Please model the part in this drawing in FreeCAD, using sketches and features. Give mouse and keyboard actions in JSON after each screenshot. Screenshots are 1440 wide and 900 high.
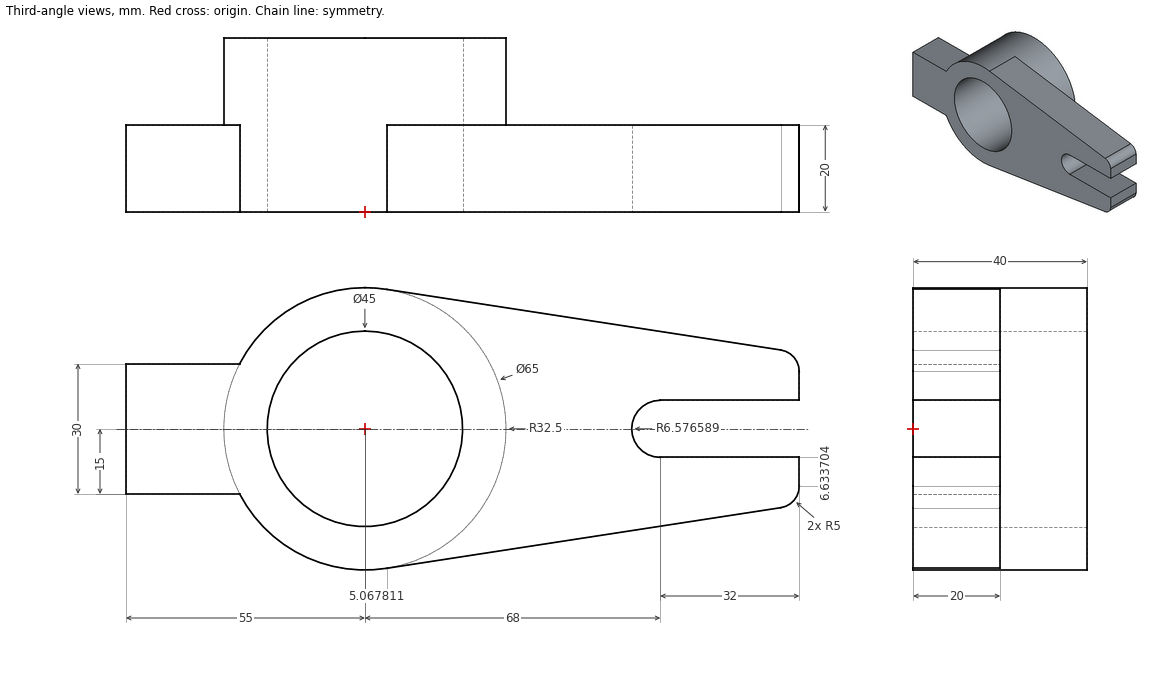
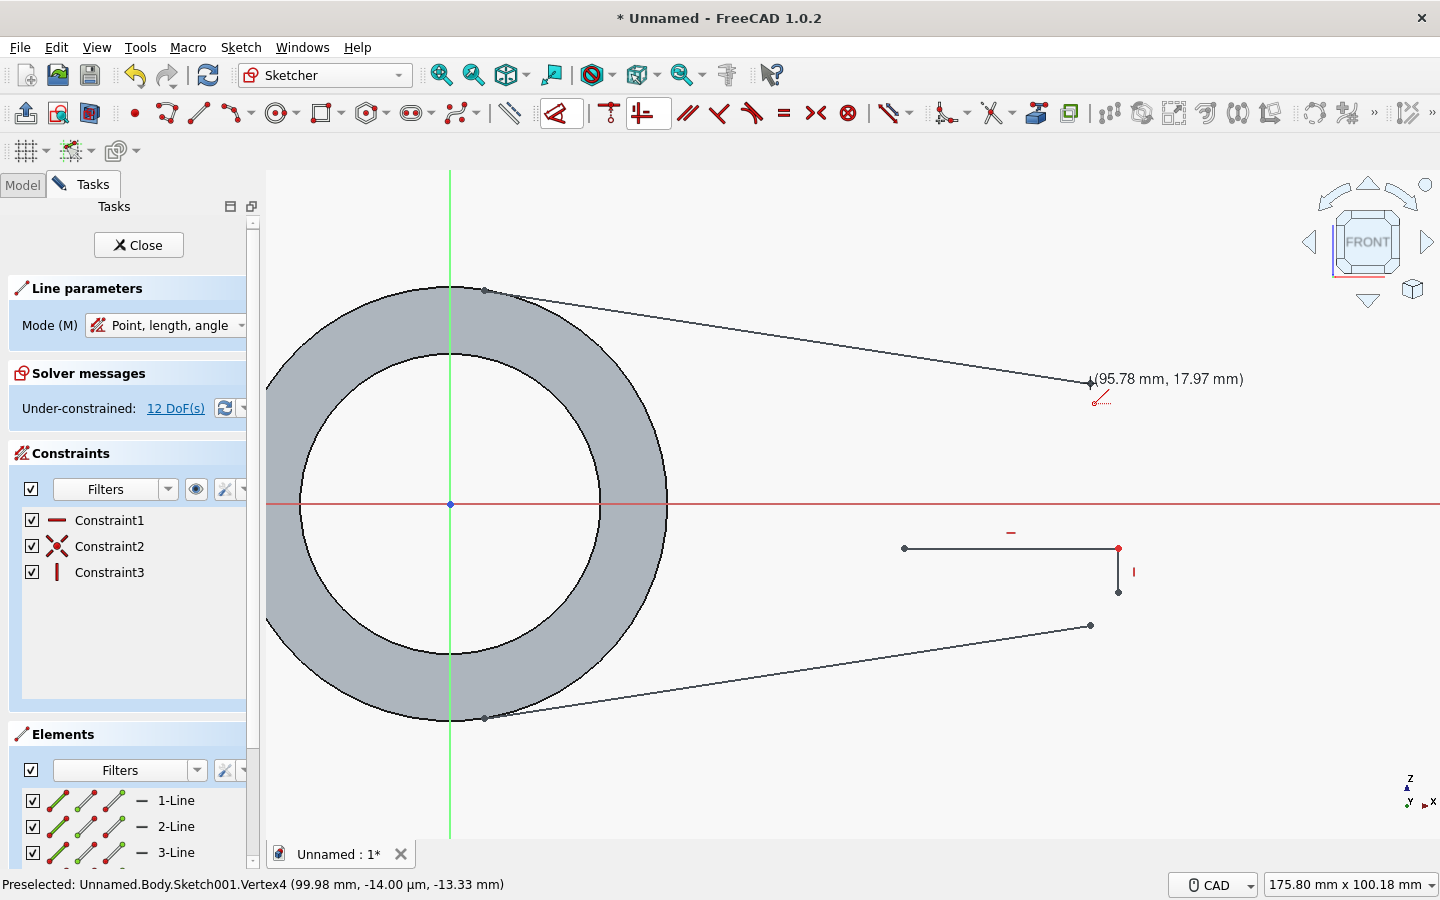
{"action": "left_click", "coordinate": [168, 114]}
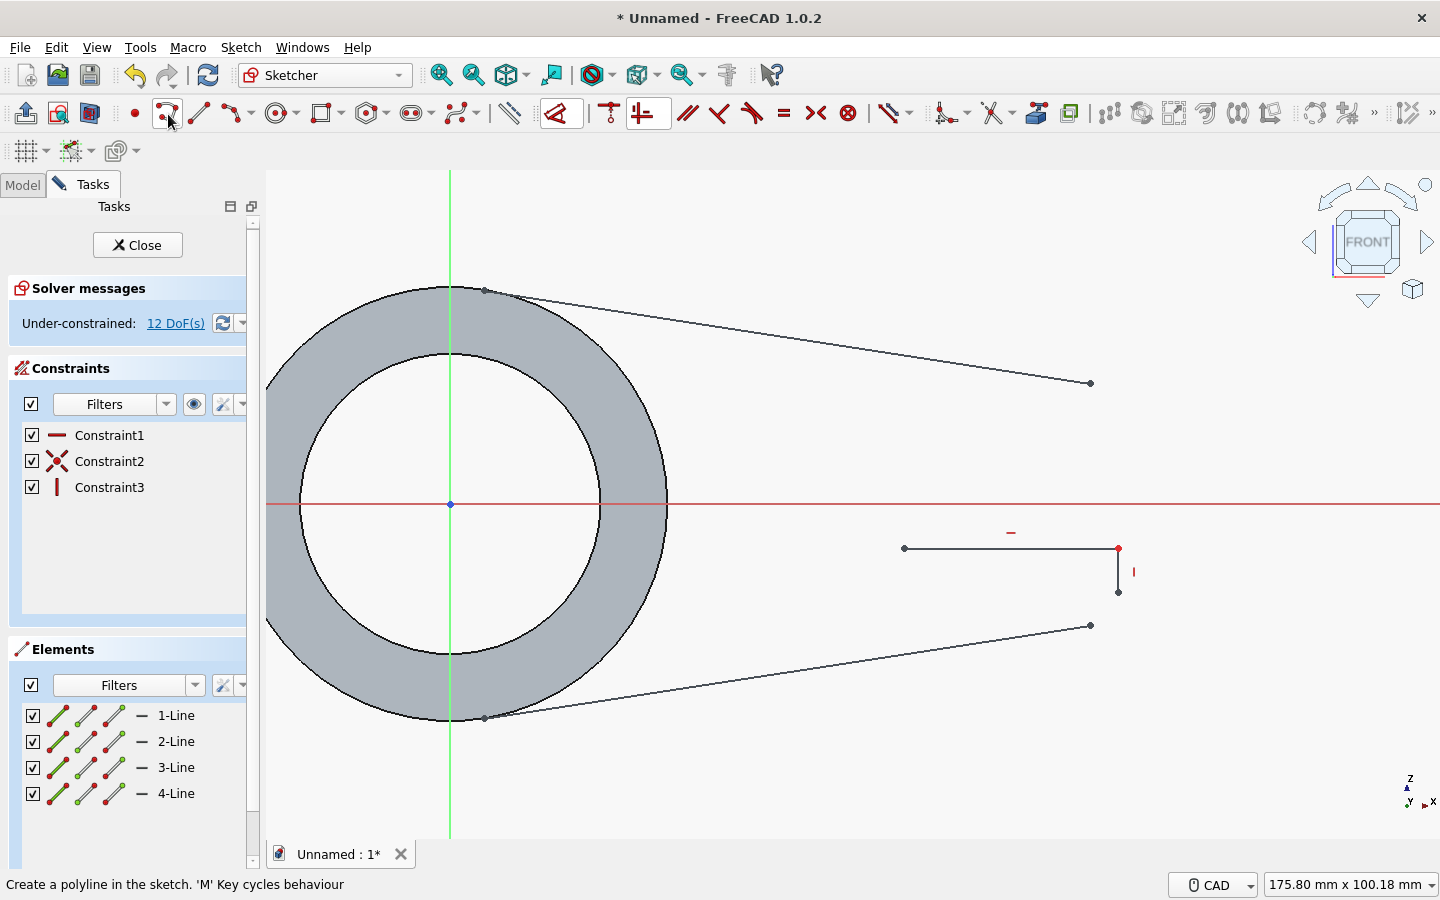
{"action": "left_click", "coordinate": [1118, 416]}
{"action": "left_click", "coordinate": [1118, 460]}
{"action": "left_click", "coordinate": [904, 460]}
{"action": "right_click", "coordinate": [904, 460]}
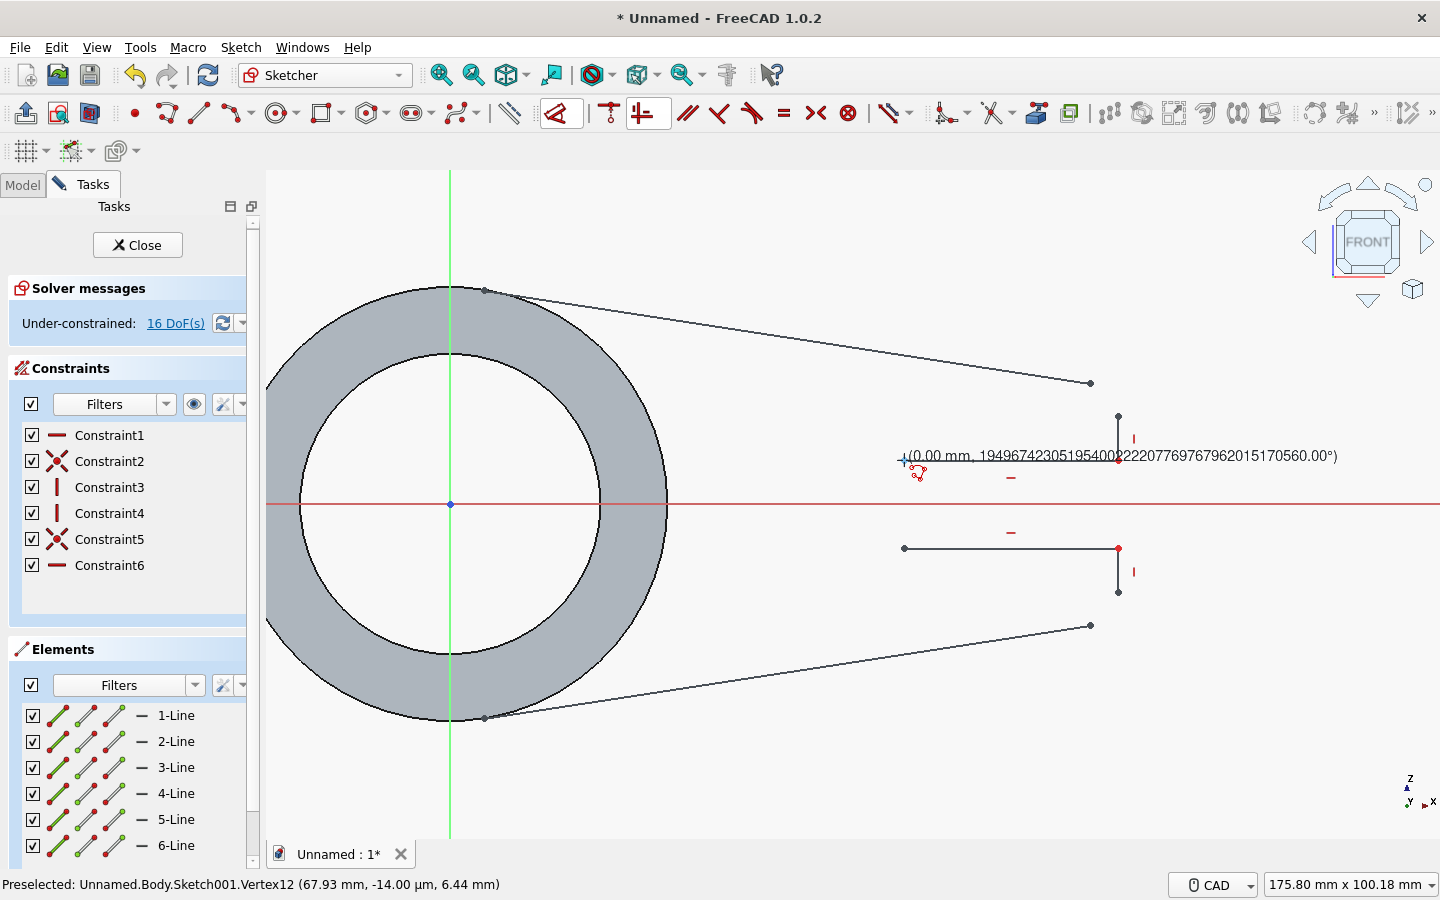
{"action": "left_click", "coordinate": [232, 114]}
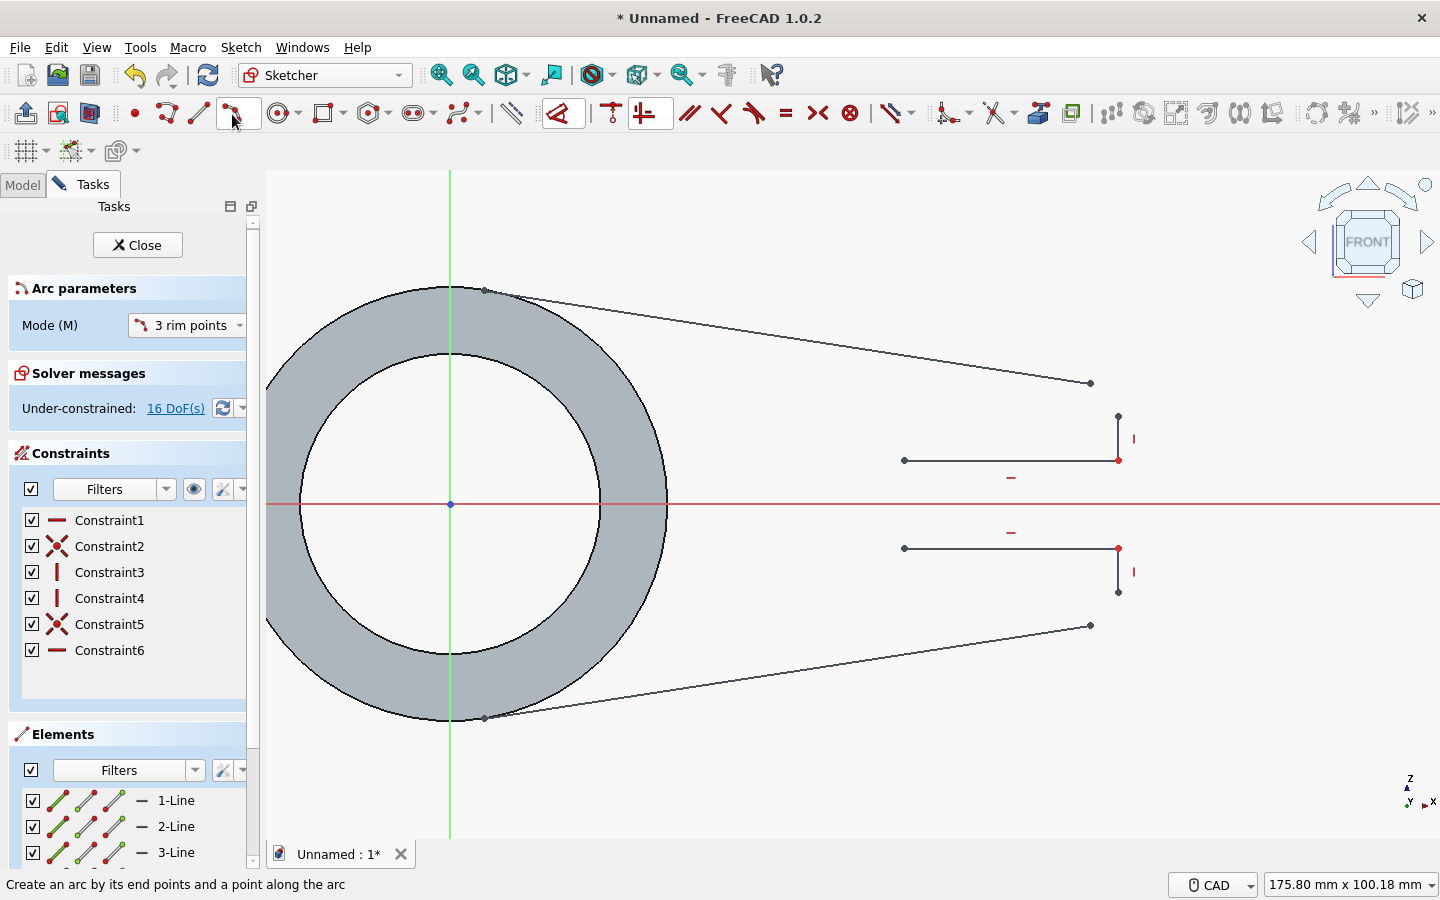
{"action": "left_click", "coordinate": [1118, 593]}
{"action": "left_click", "coordinate": [1090, 626]}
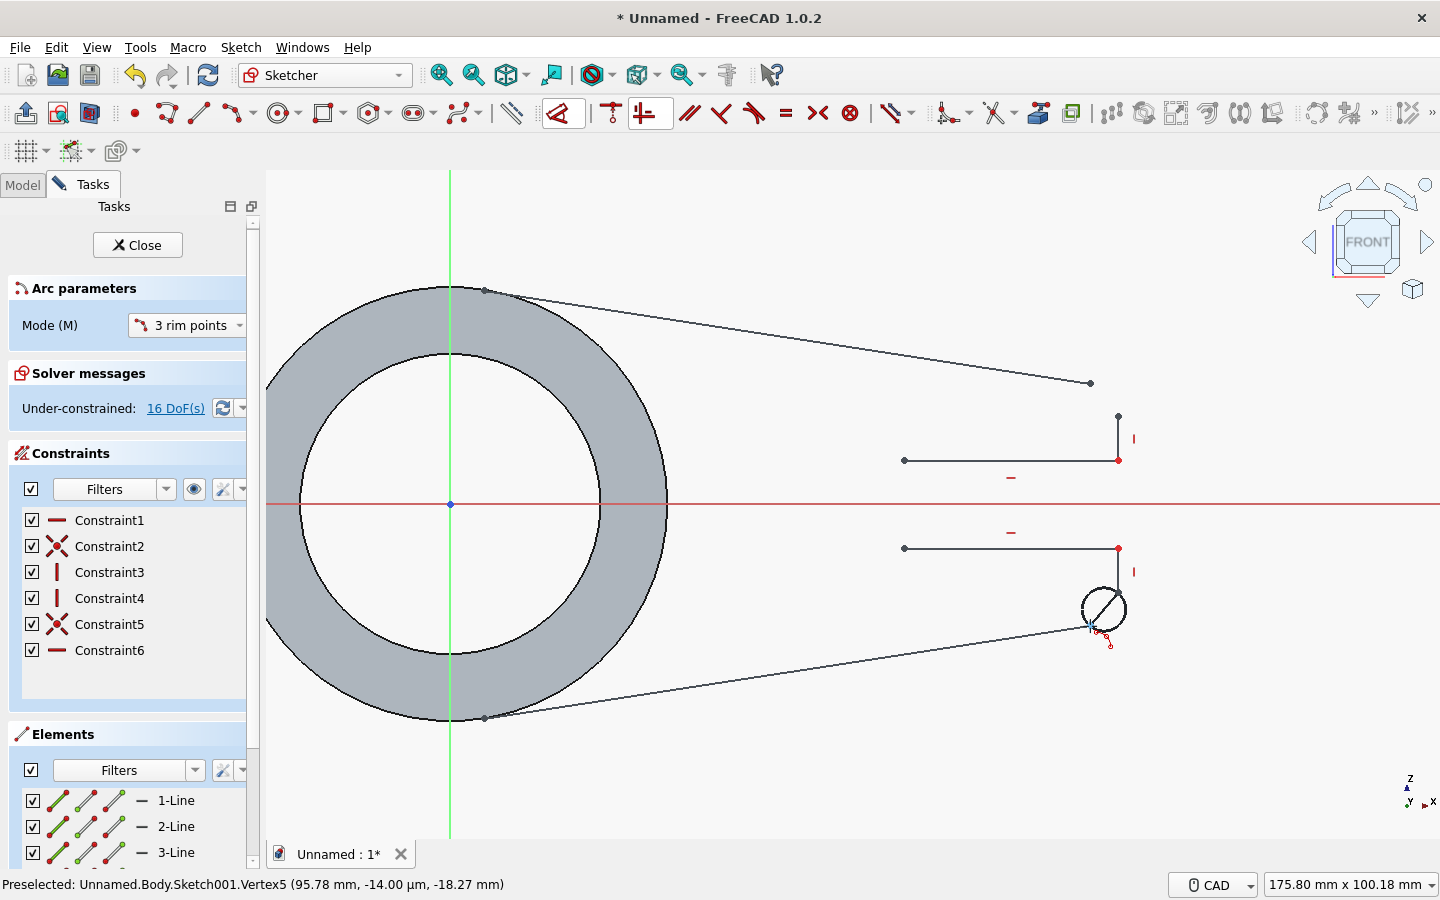
{"action": "scroll", "coordinate": [1110, 614], "scroll_direction": "up", "scroll_amount": 4}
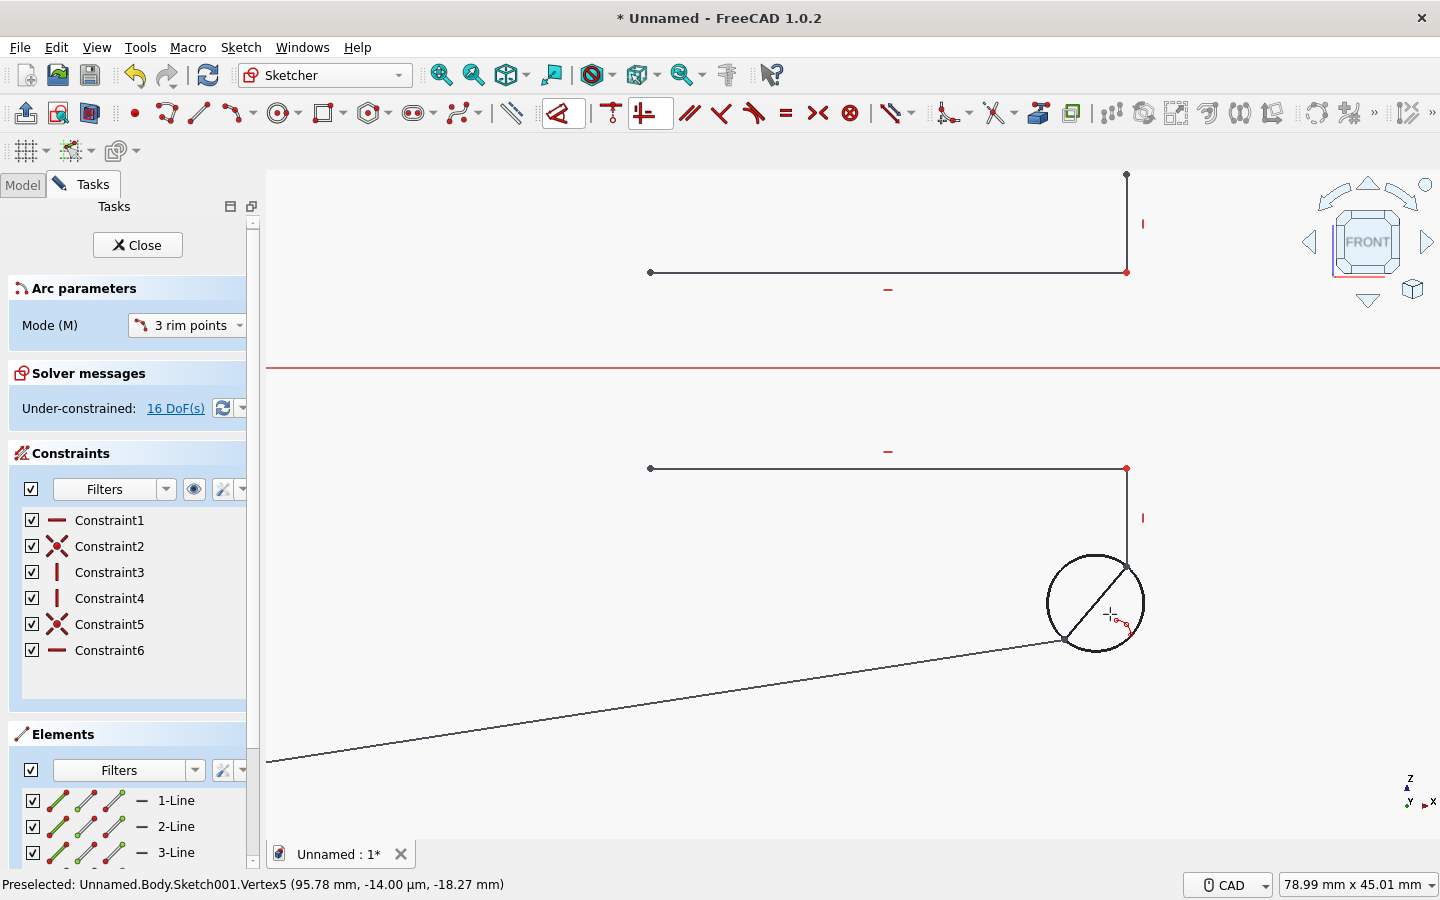
{"action": "left_click", "coordinate": [1109, 613]}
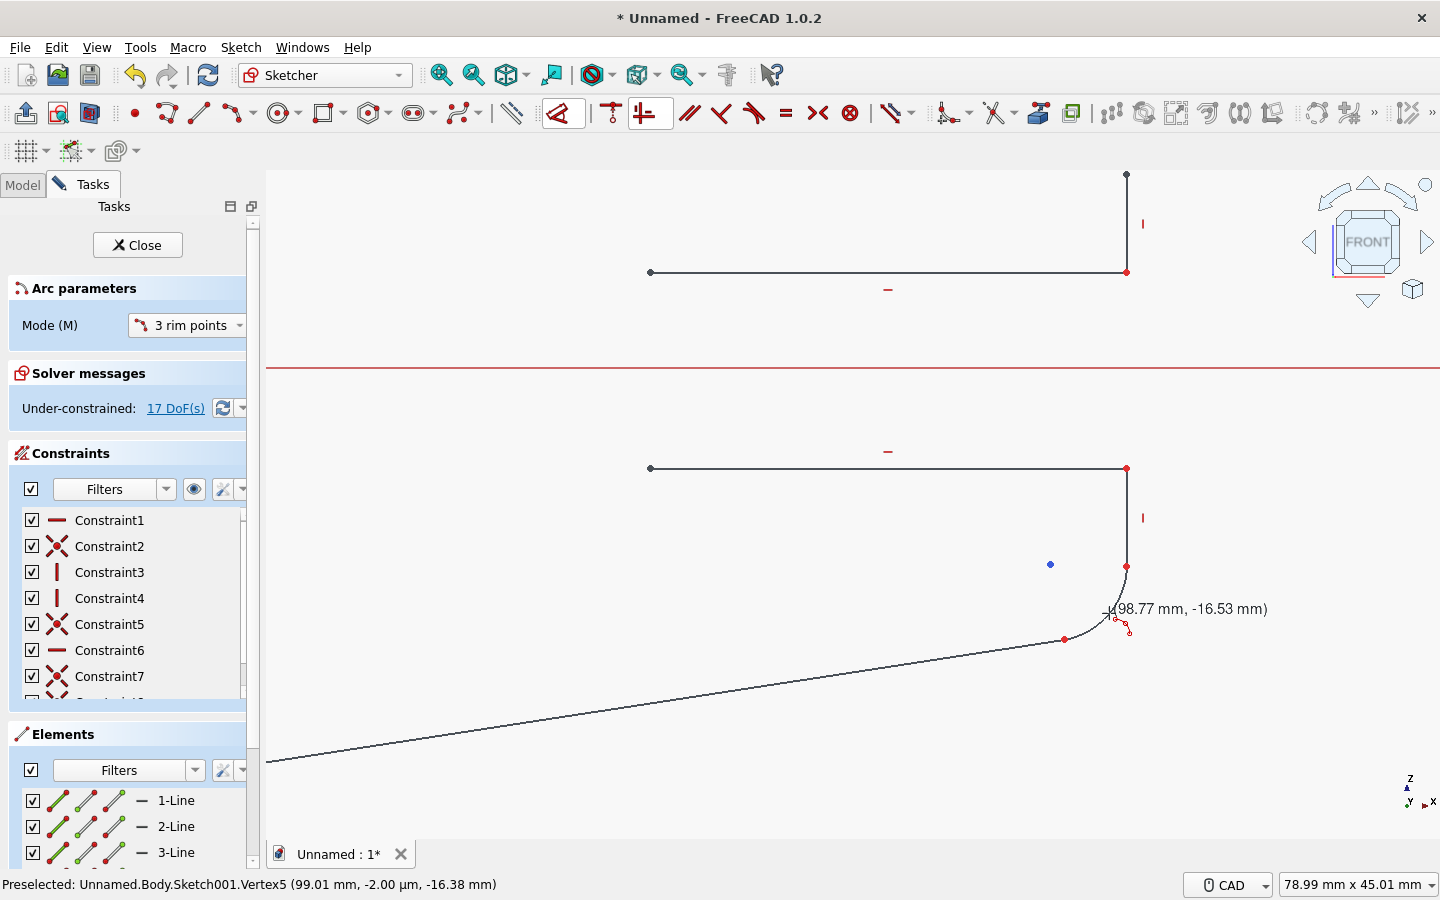
{"action": "scroll", "coordinate": [1111, 616], "scroll_direction": "down", "scroll_amount": 4}